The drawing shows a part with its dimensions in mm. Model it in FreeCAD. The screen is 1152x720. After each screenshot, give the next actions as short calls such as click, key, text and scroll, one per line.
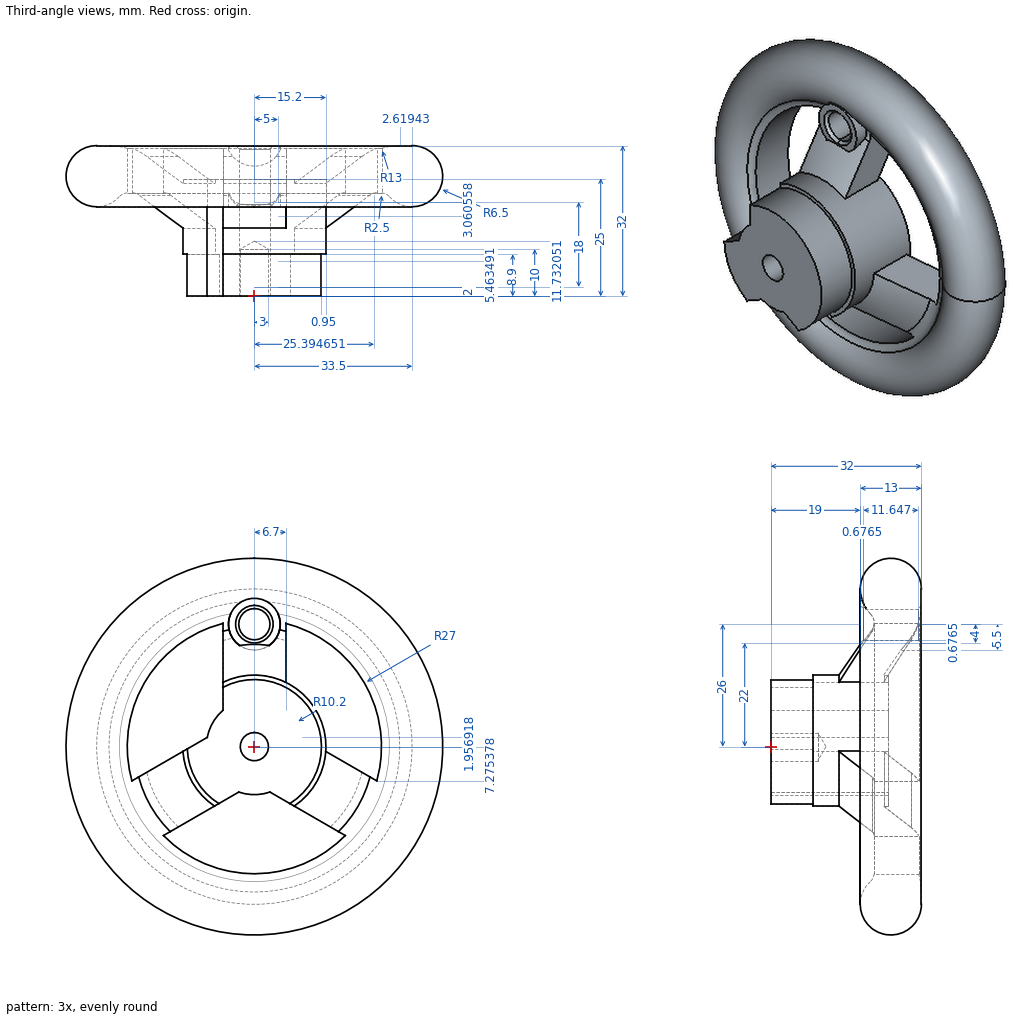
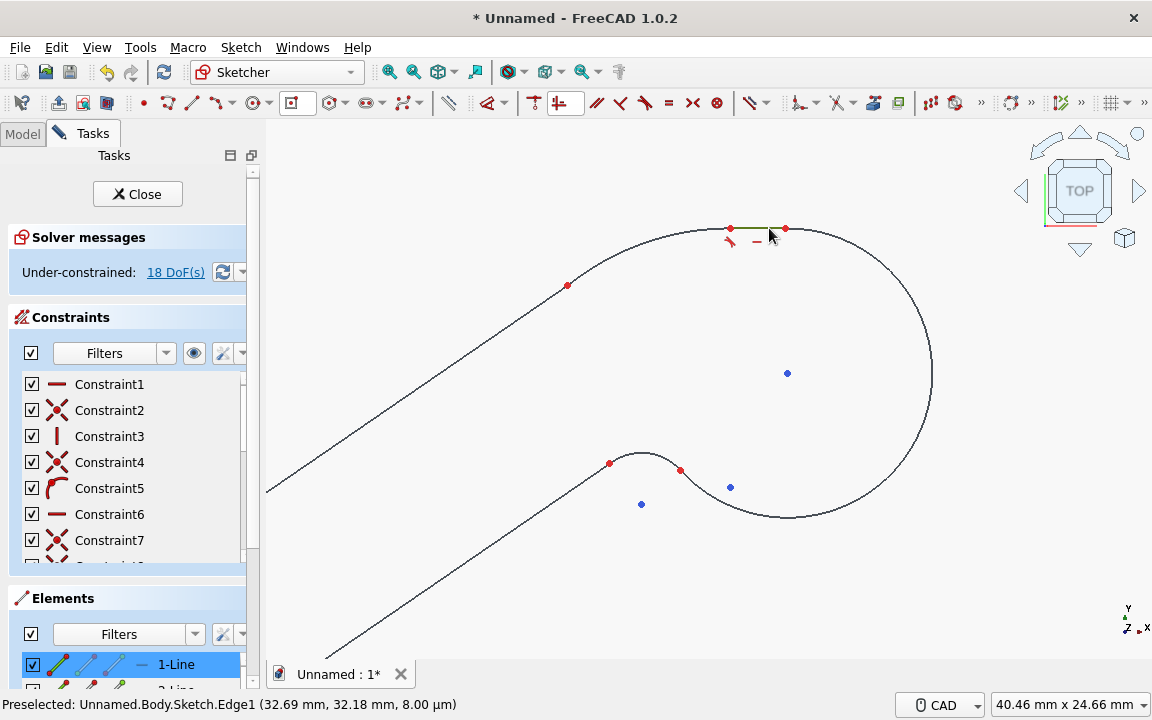
click(839, 508)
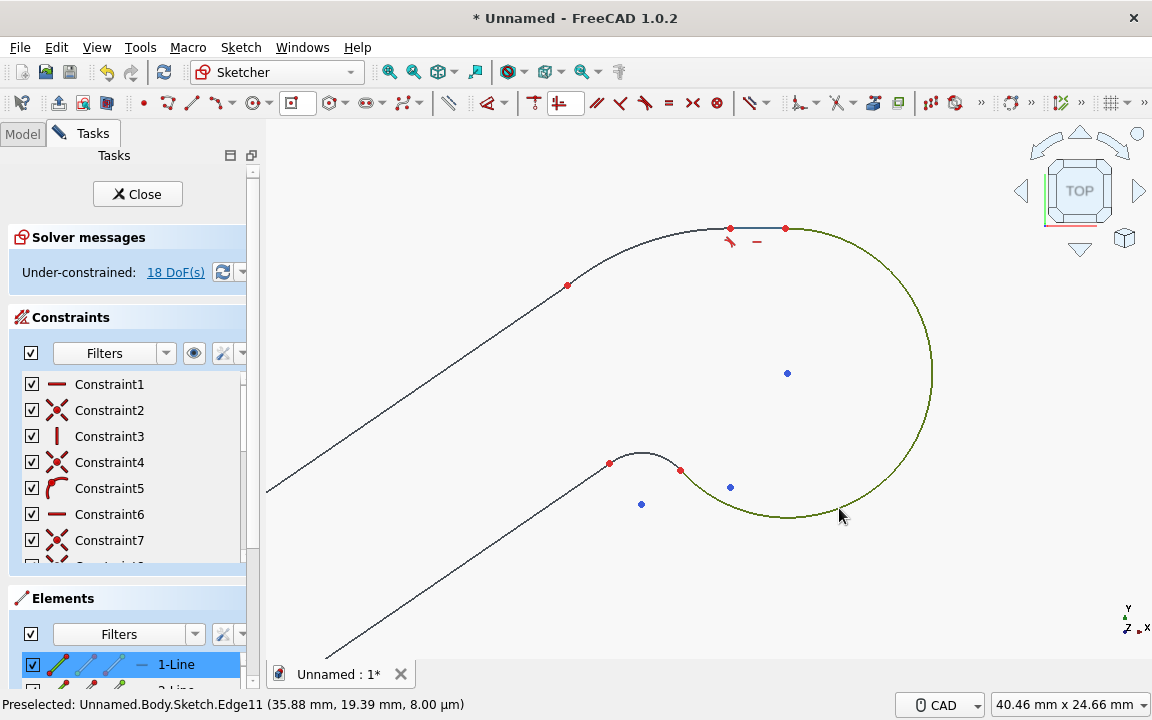
key(t)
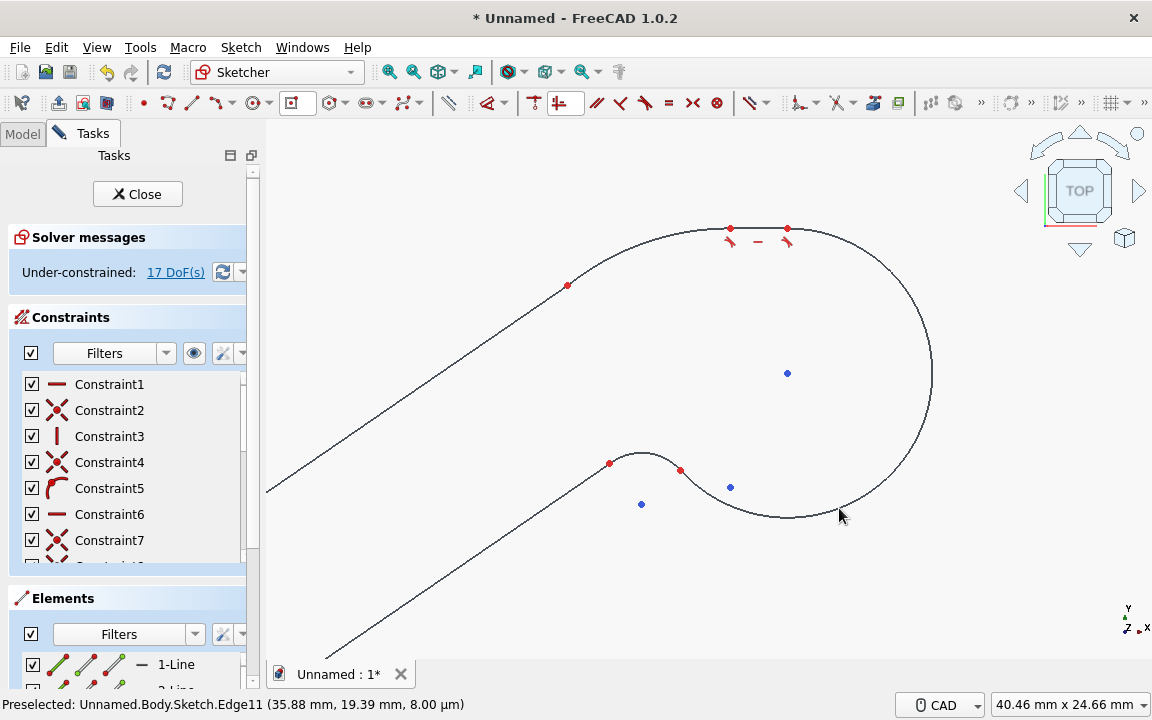
click(446, 369)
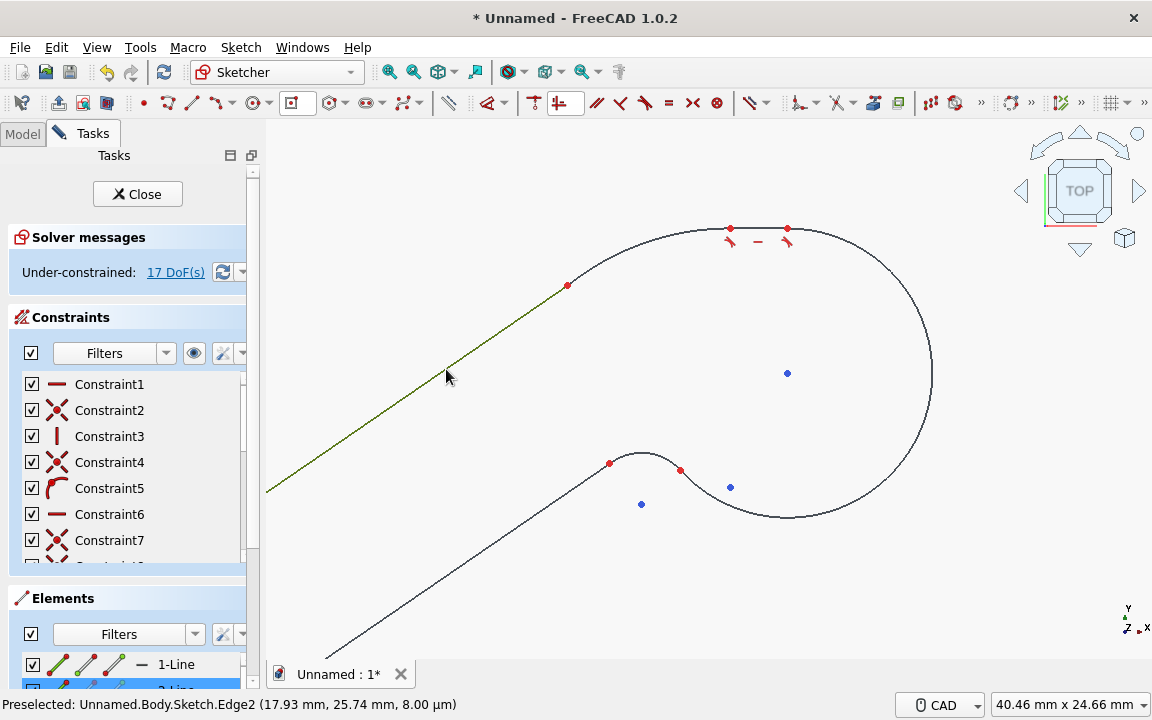
click(678, 234)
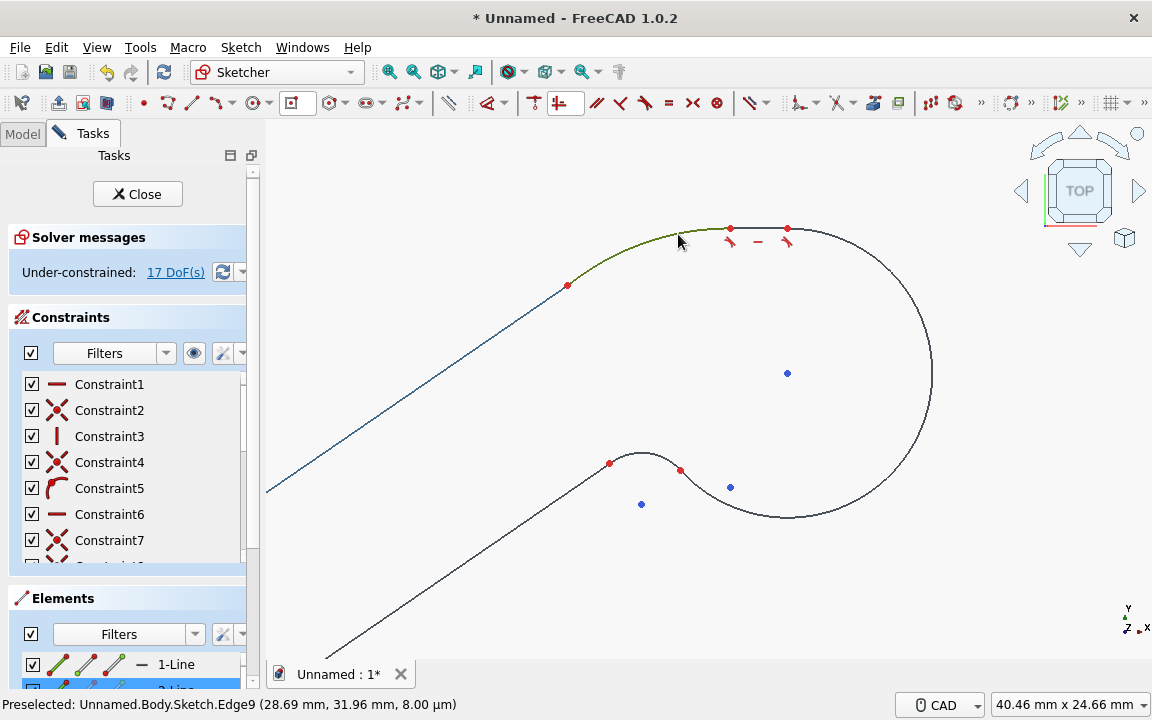
click(646, 104)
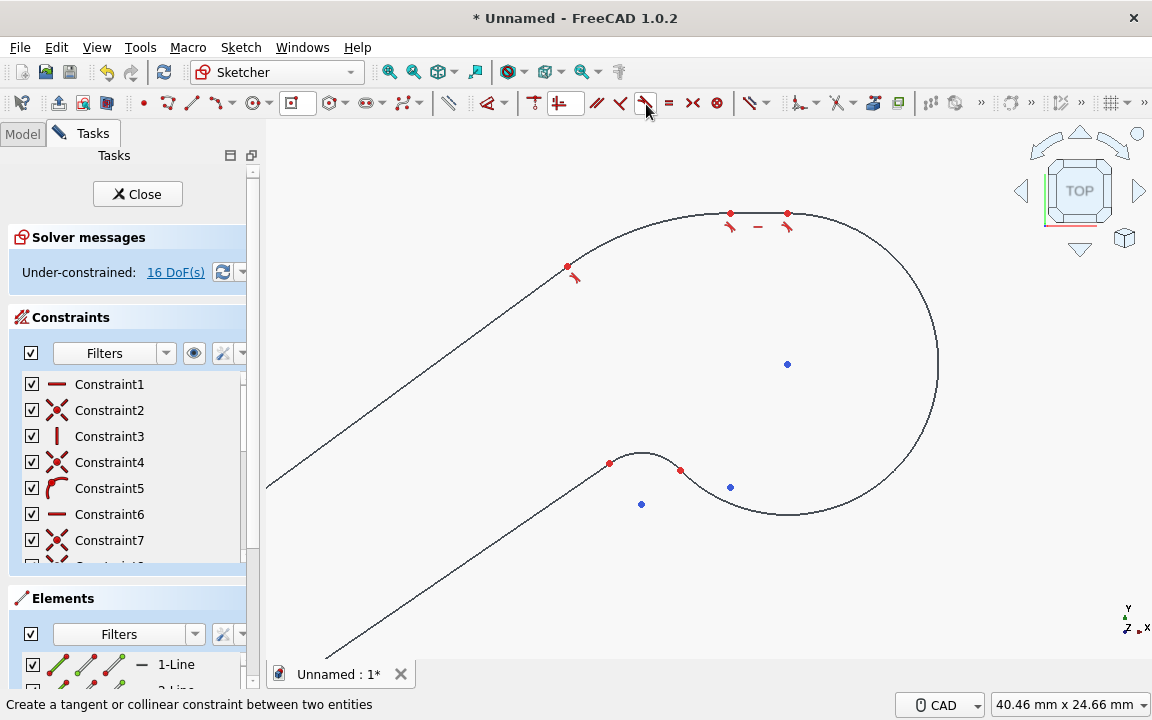
click(476, 556)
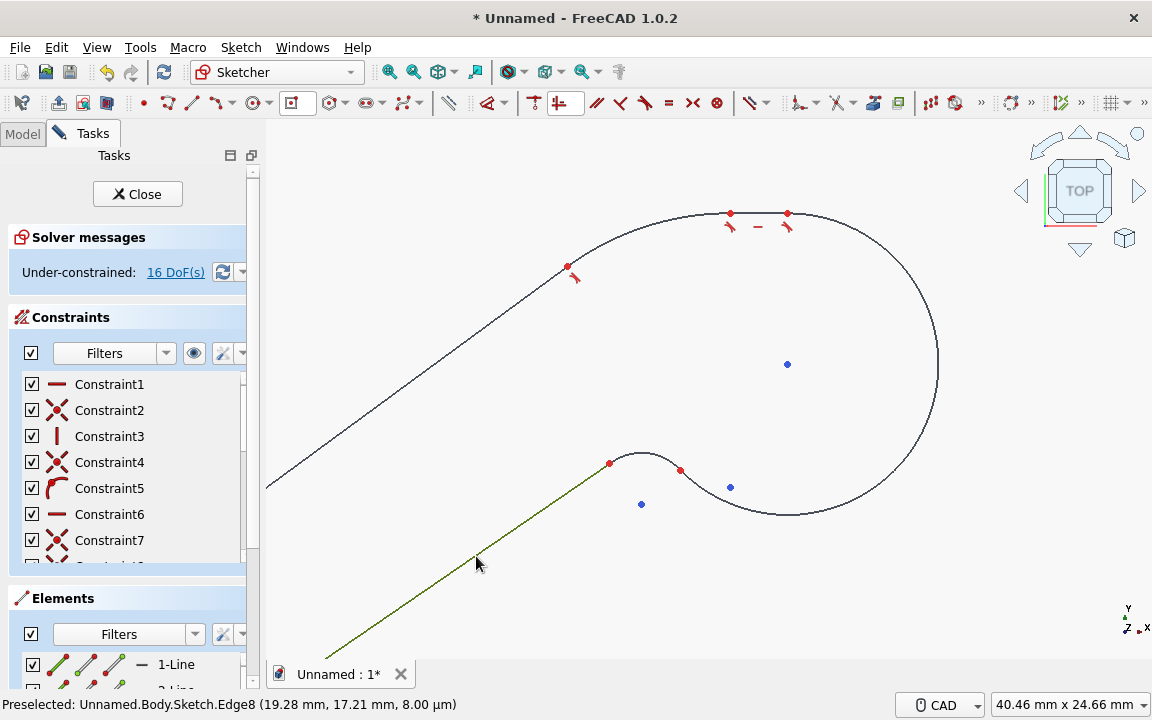
click(662, 457)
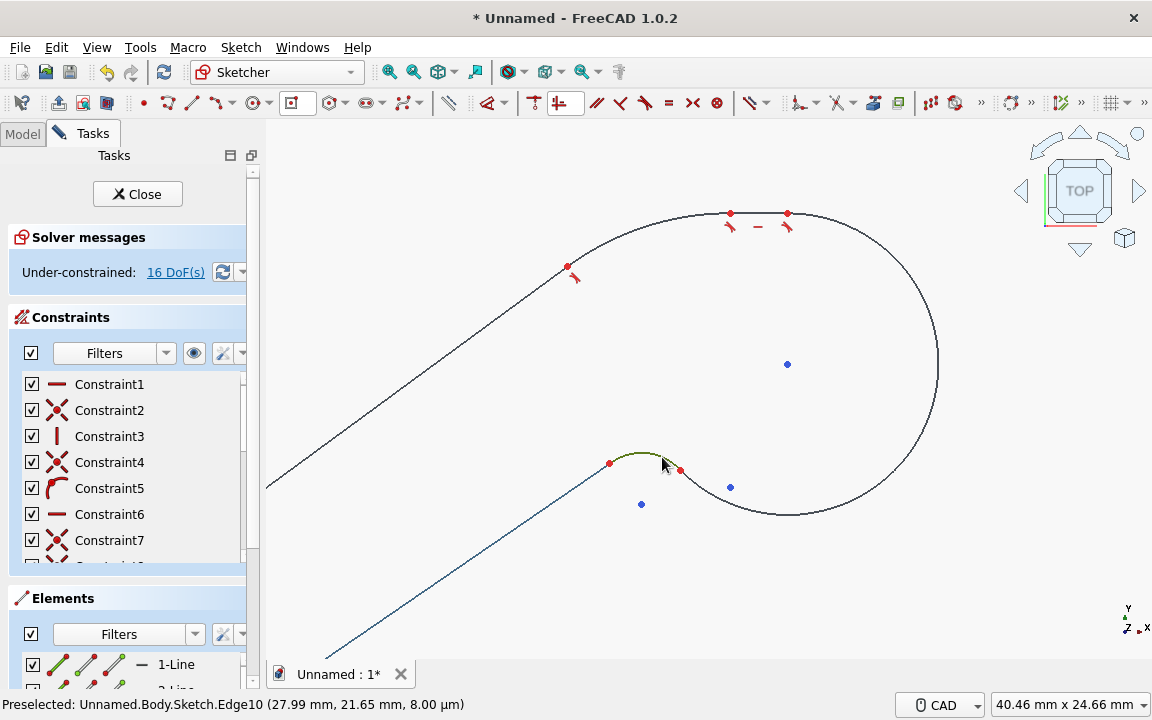
key(t)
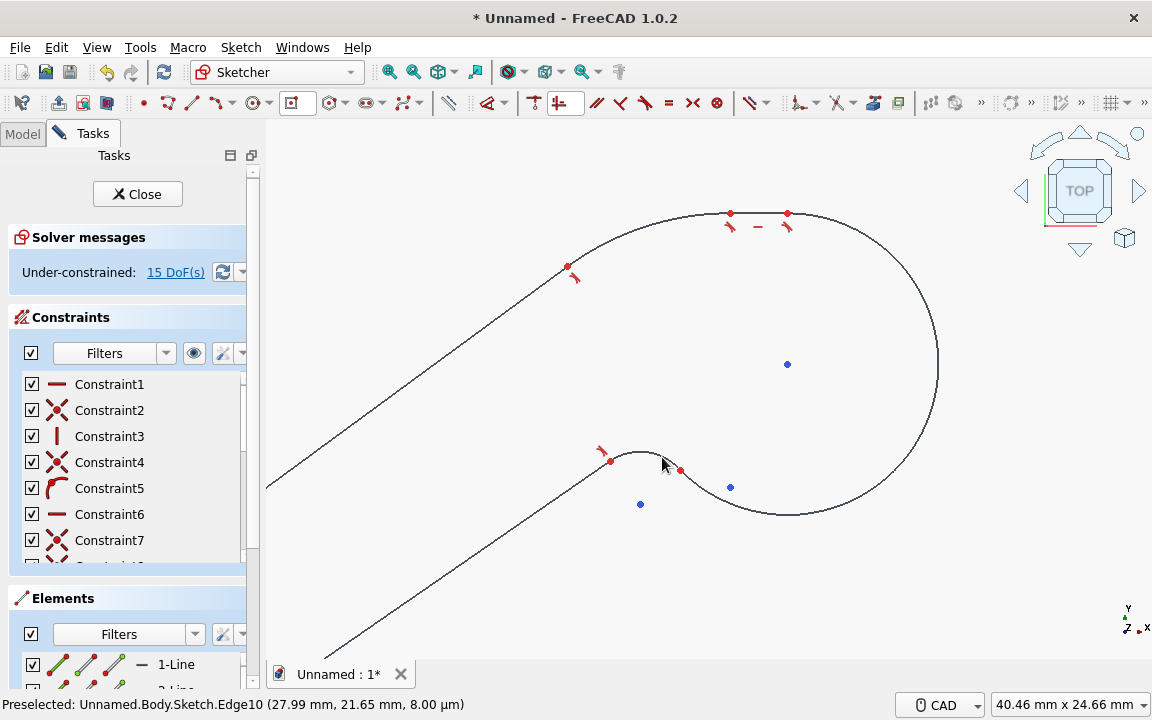
click(662, 457)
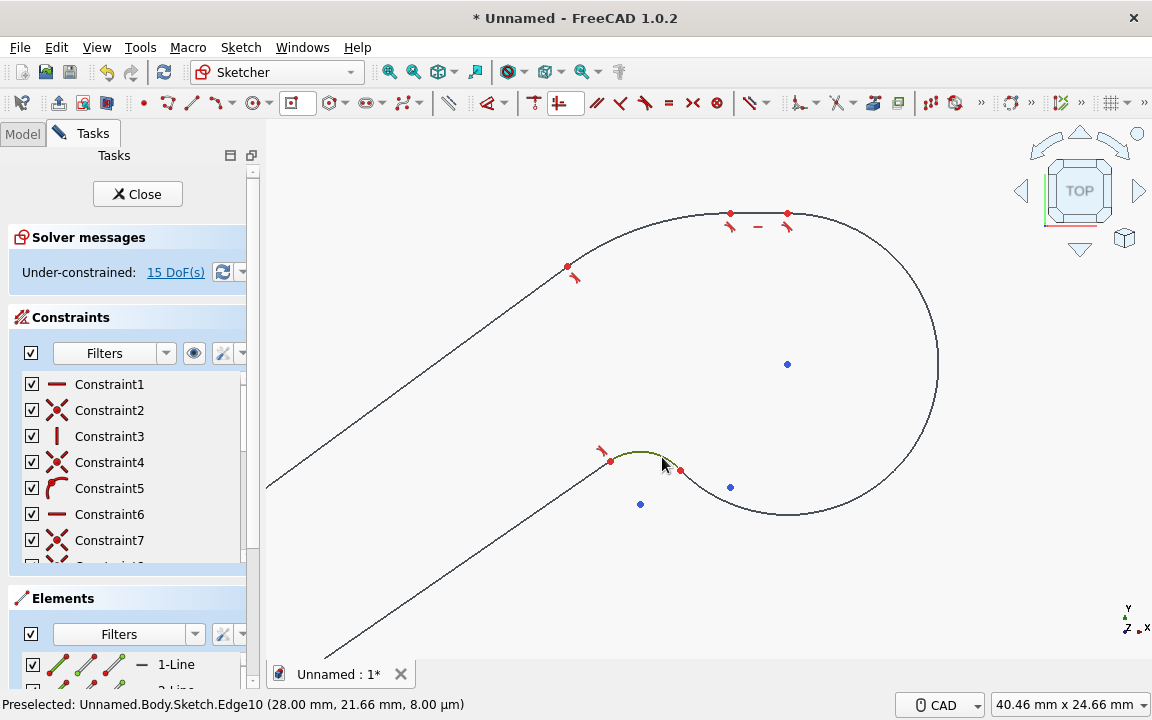
click(845, 504)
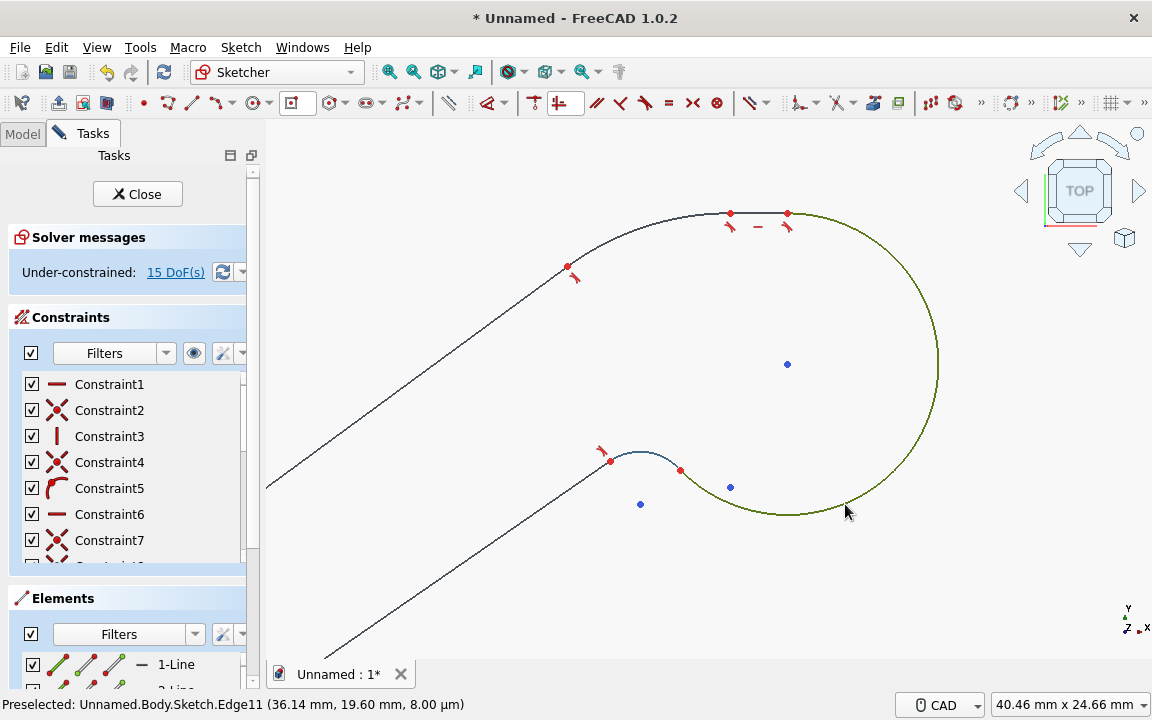
click(646, 104)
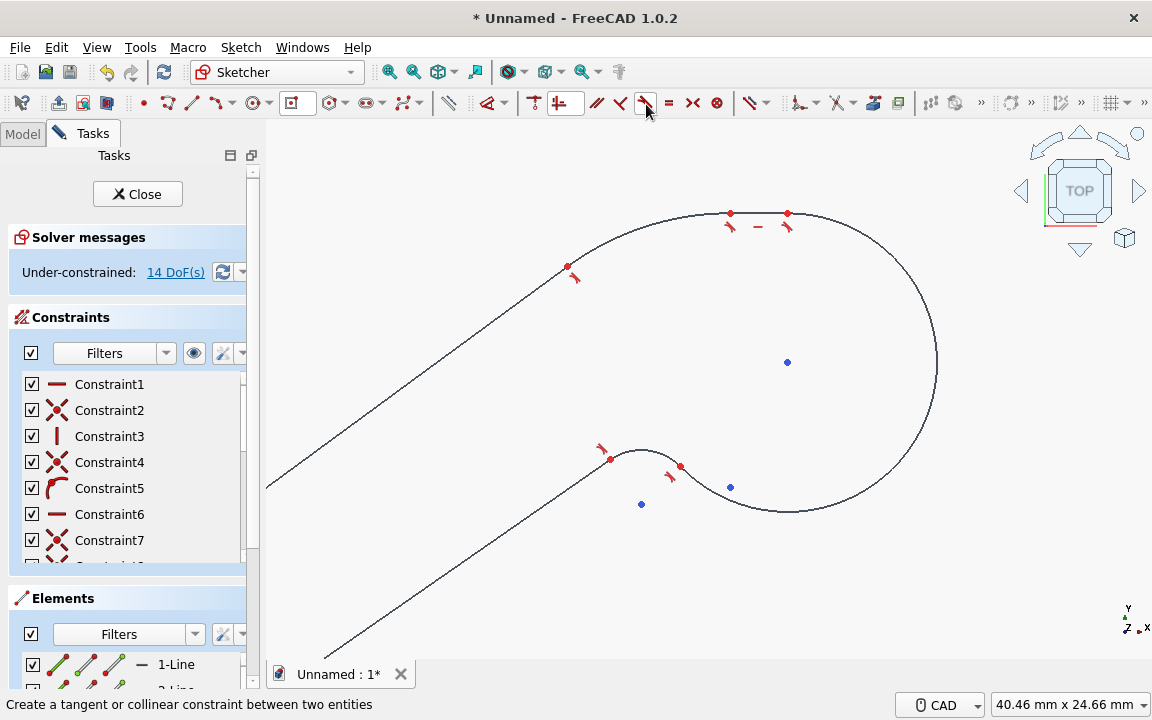
scroll(767, 231, down, 4)